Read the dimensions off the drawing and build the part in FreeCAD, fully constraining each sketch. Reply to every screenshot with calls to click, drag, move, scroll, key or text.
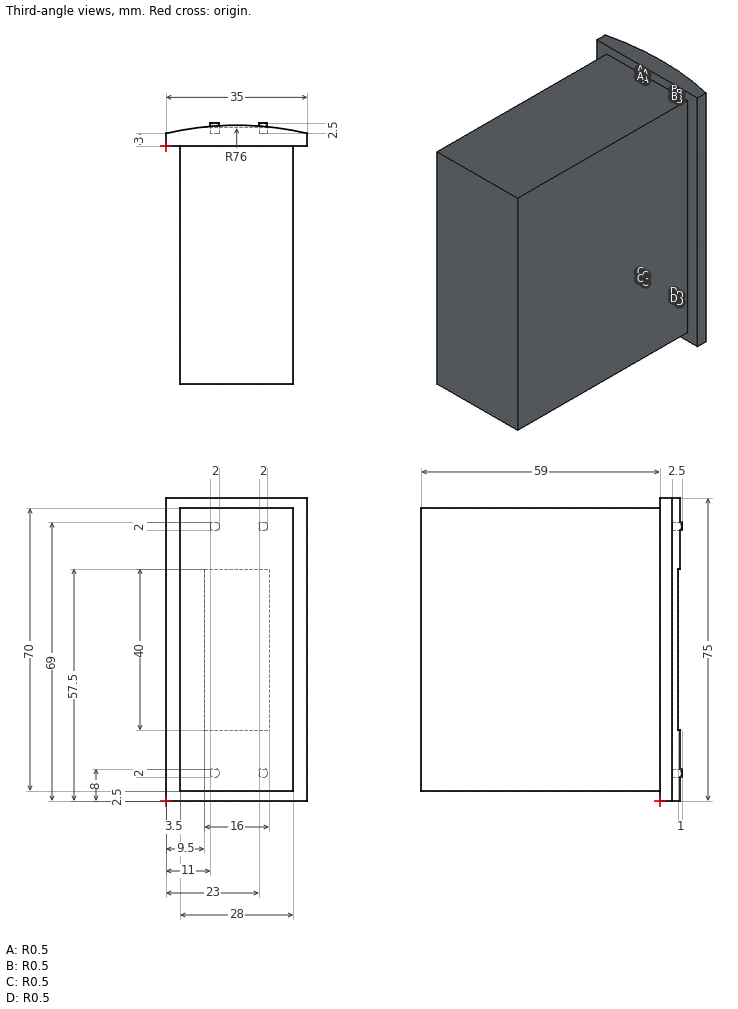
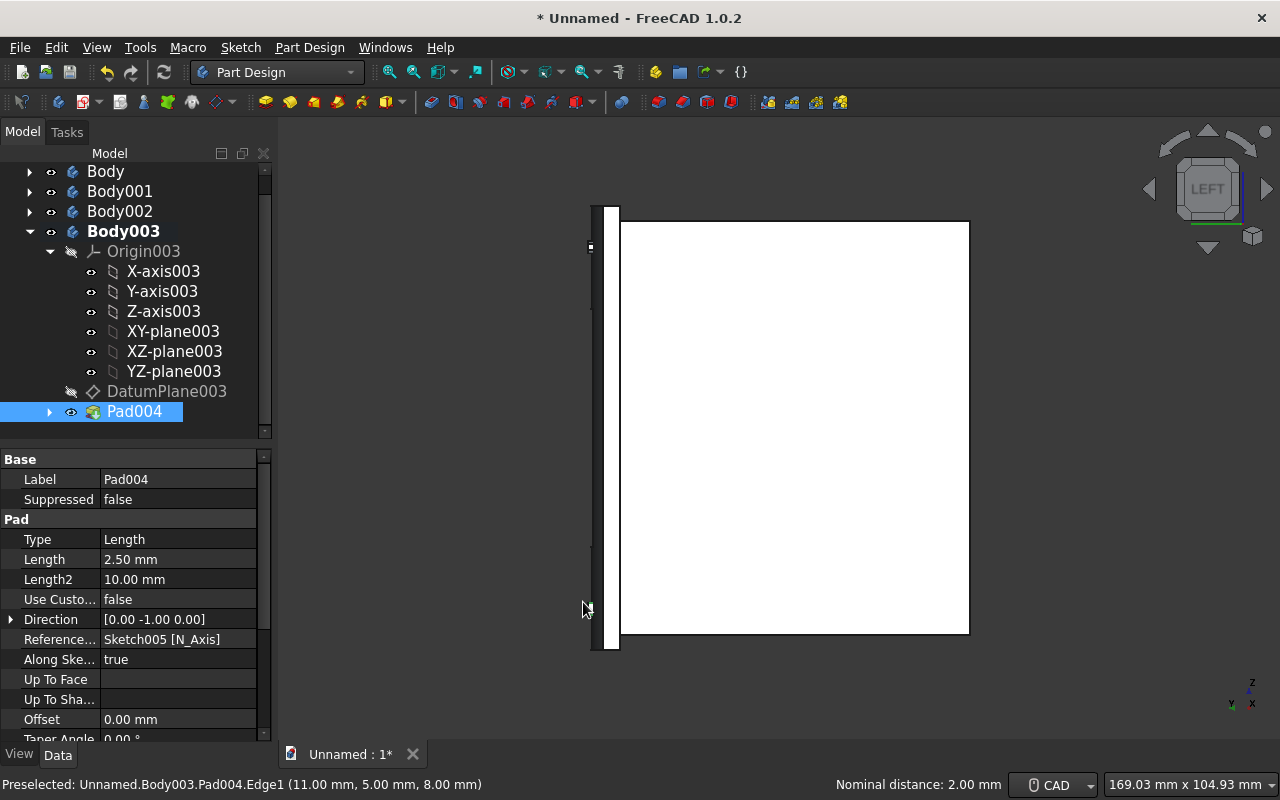
key(v)
key(3)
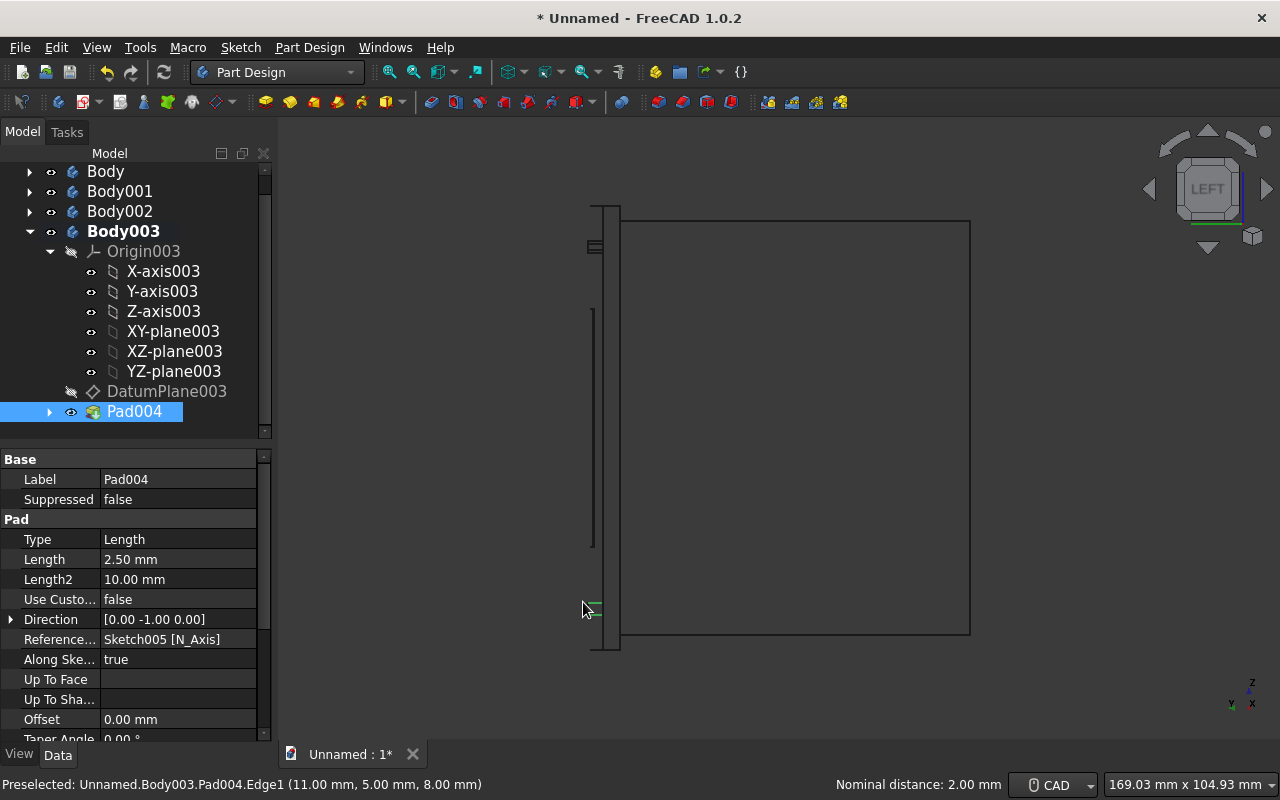
key(0)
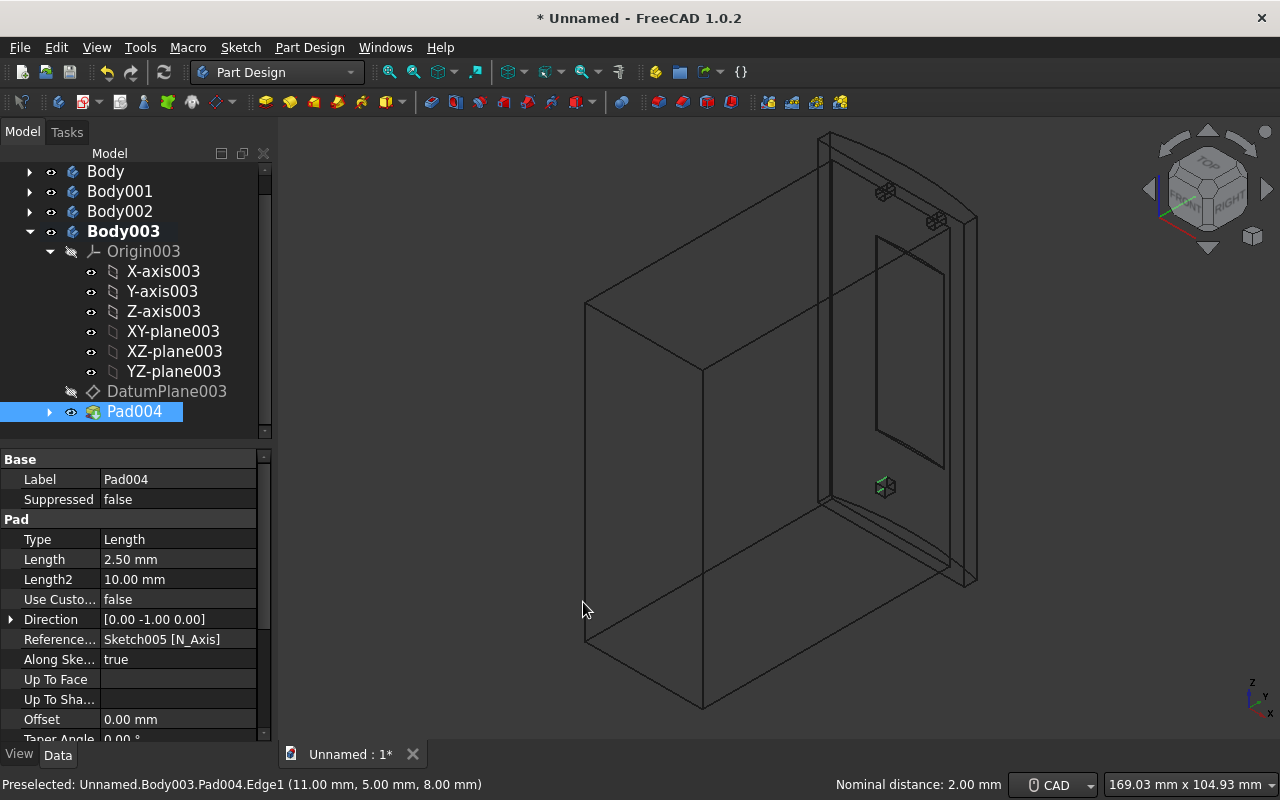
click(390, 72)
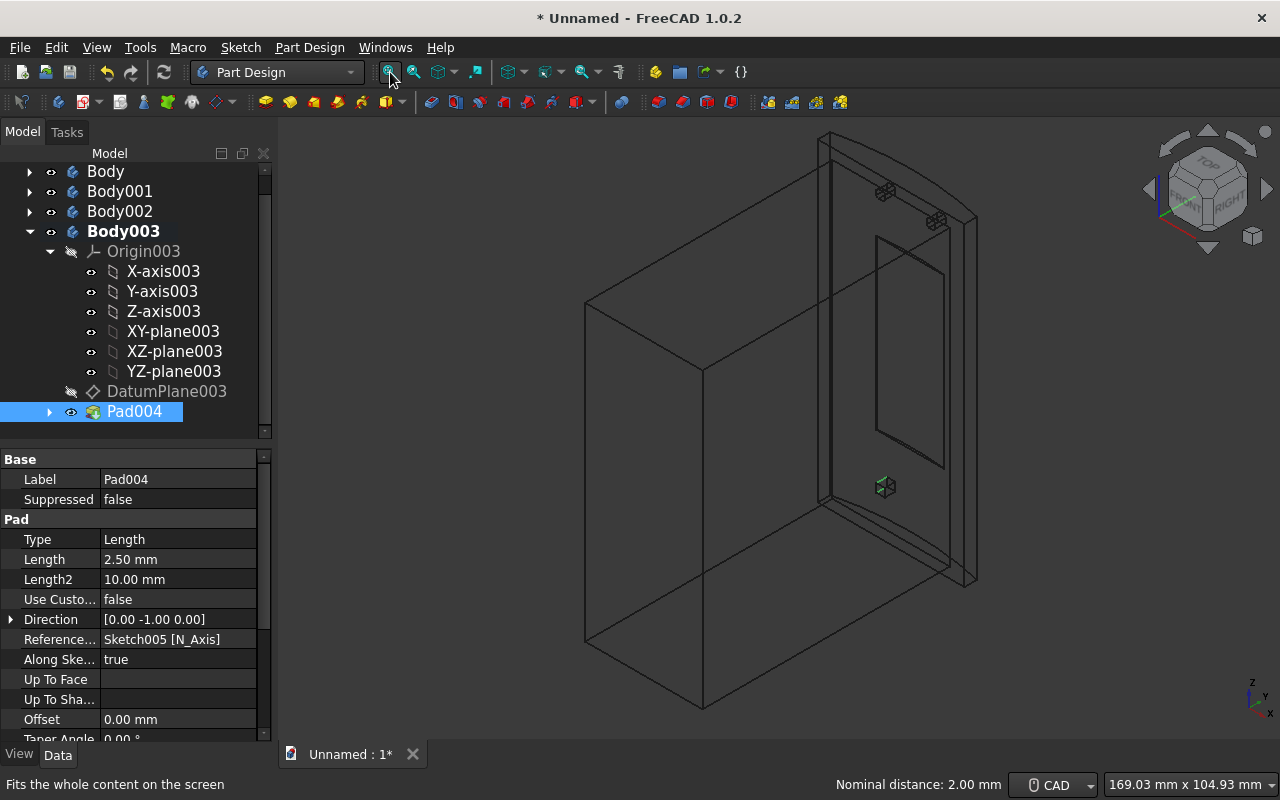
click(891, 483, ctrl)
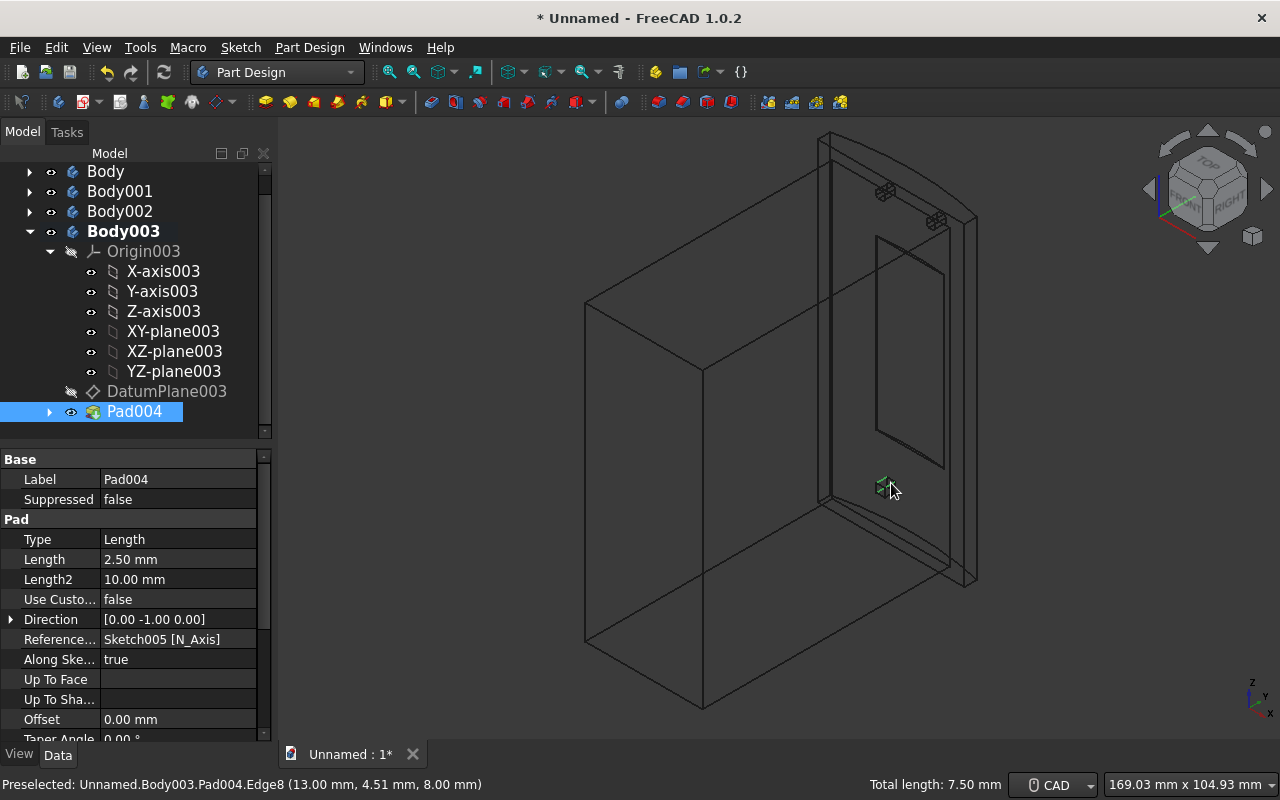
click(891, 493, ctrl)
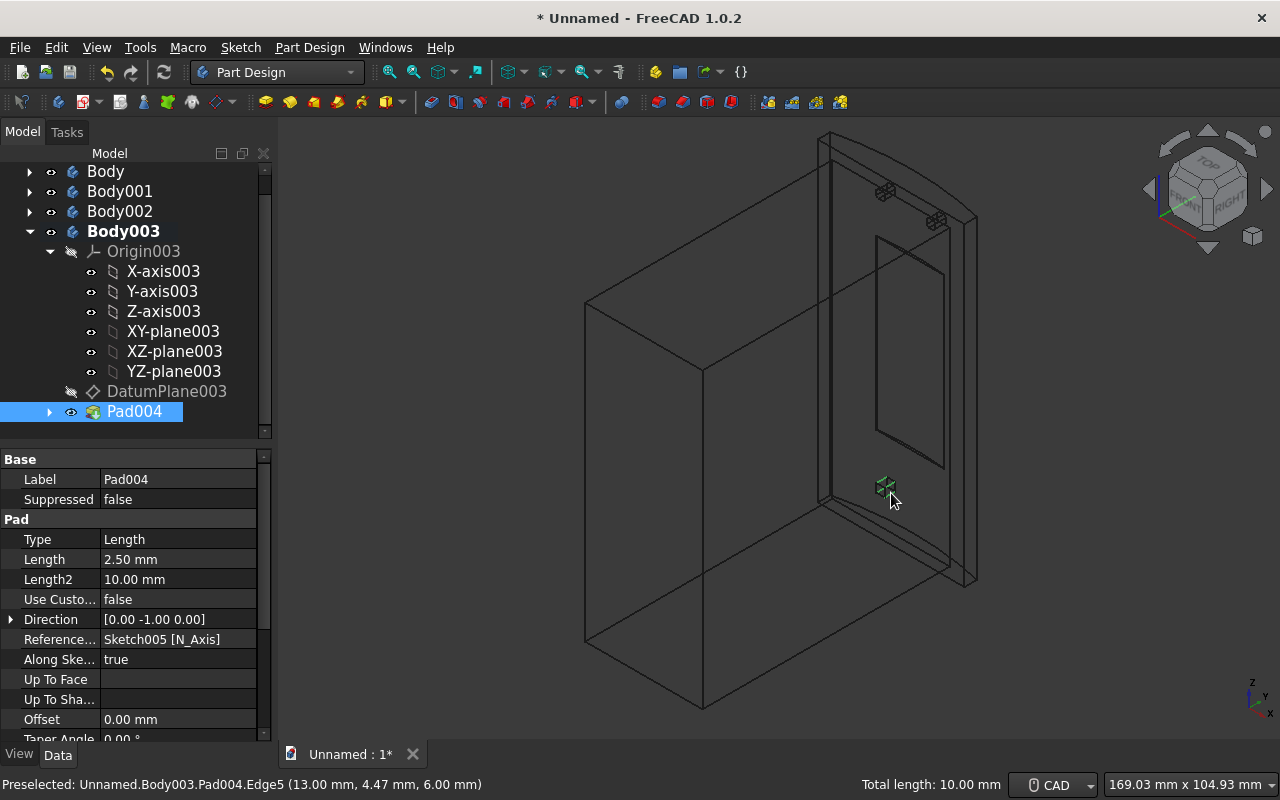
key(v)
key(1)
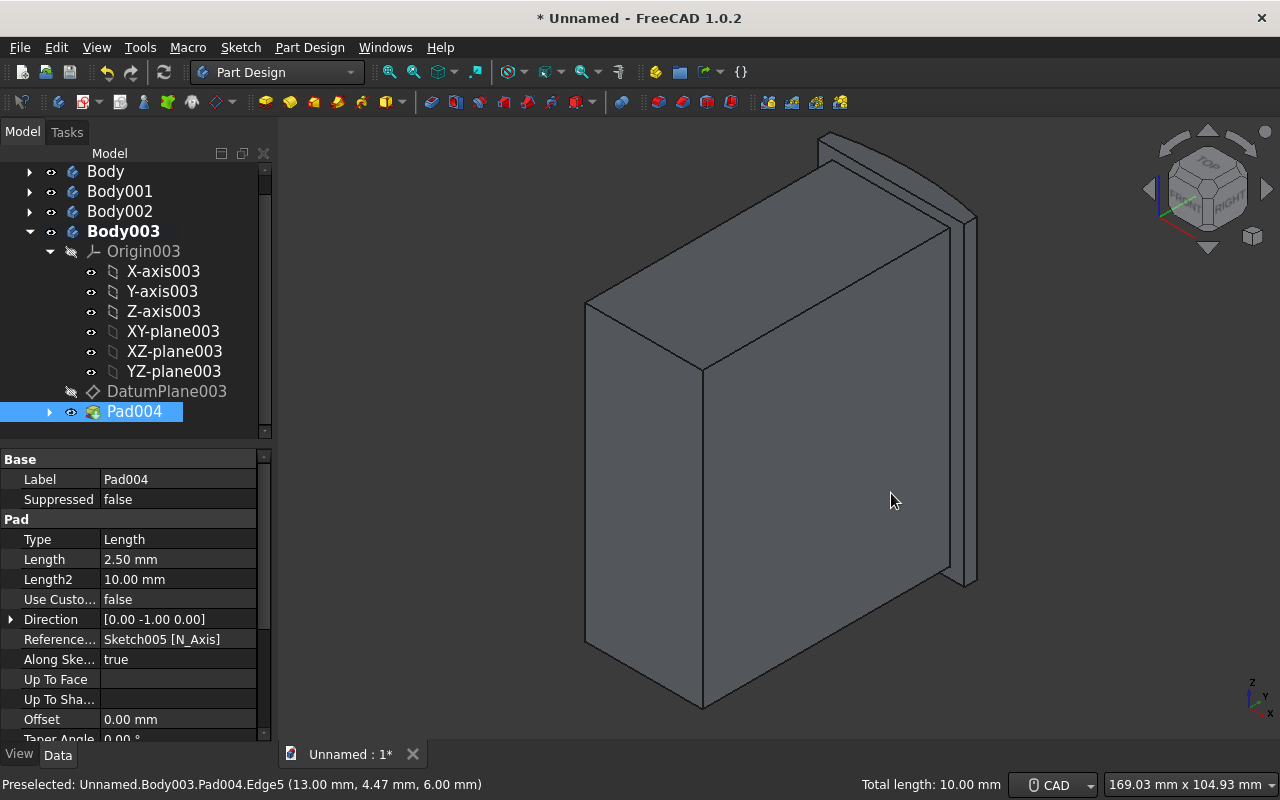
click(660, 102)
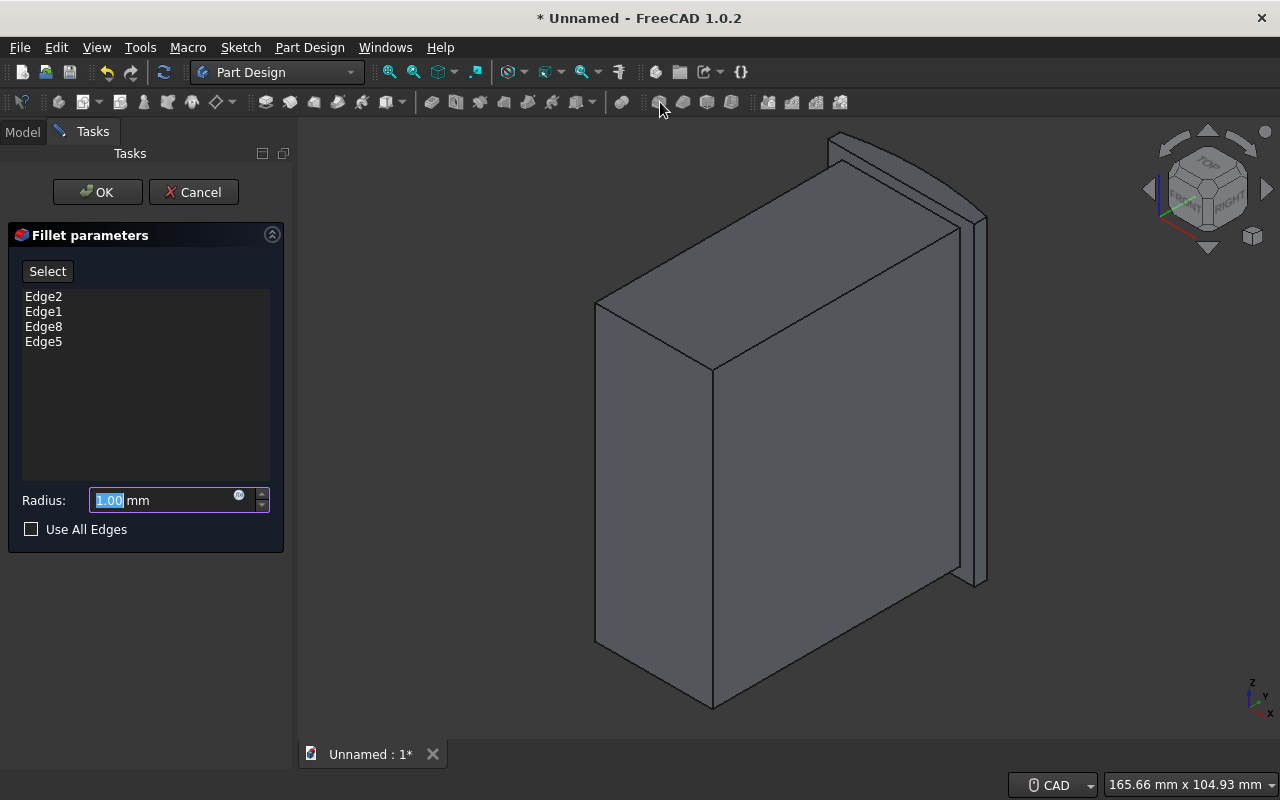
text(0.5)
key(Tab)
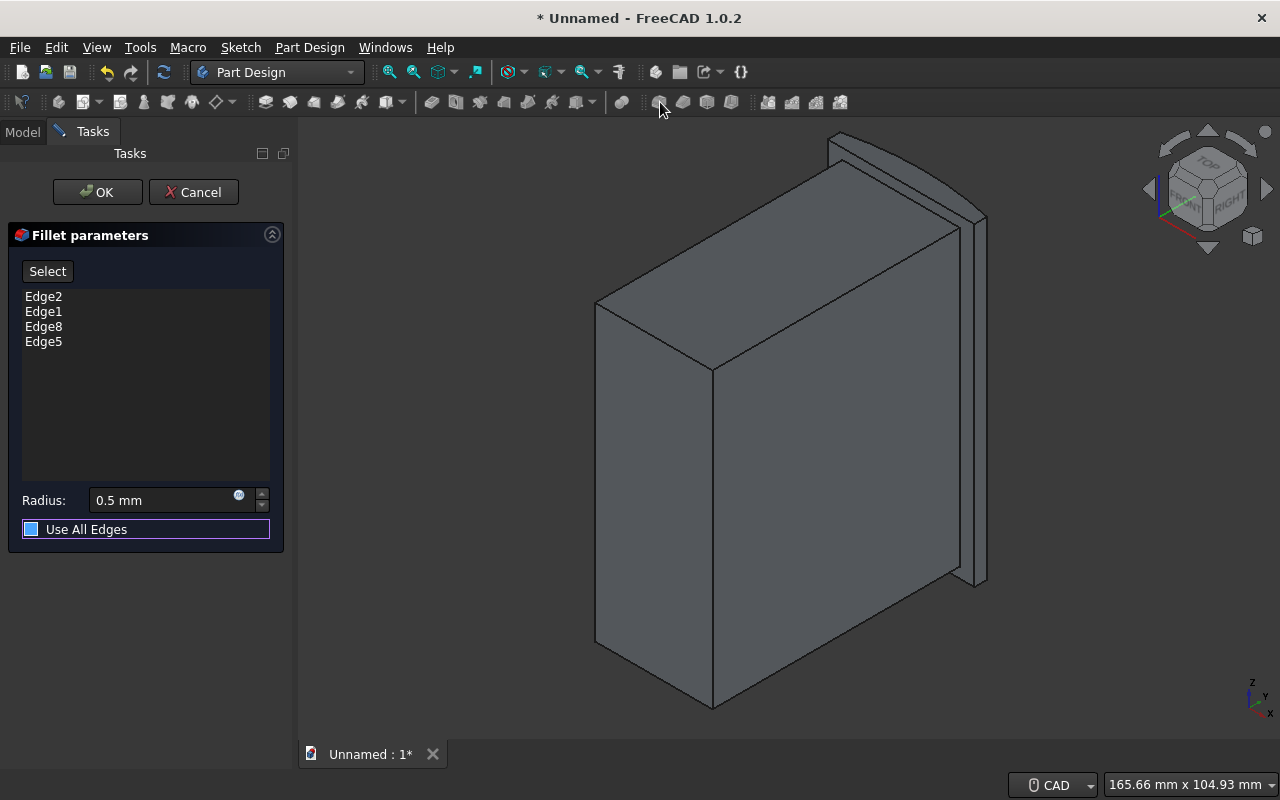
click(98, 192)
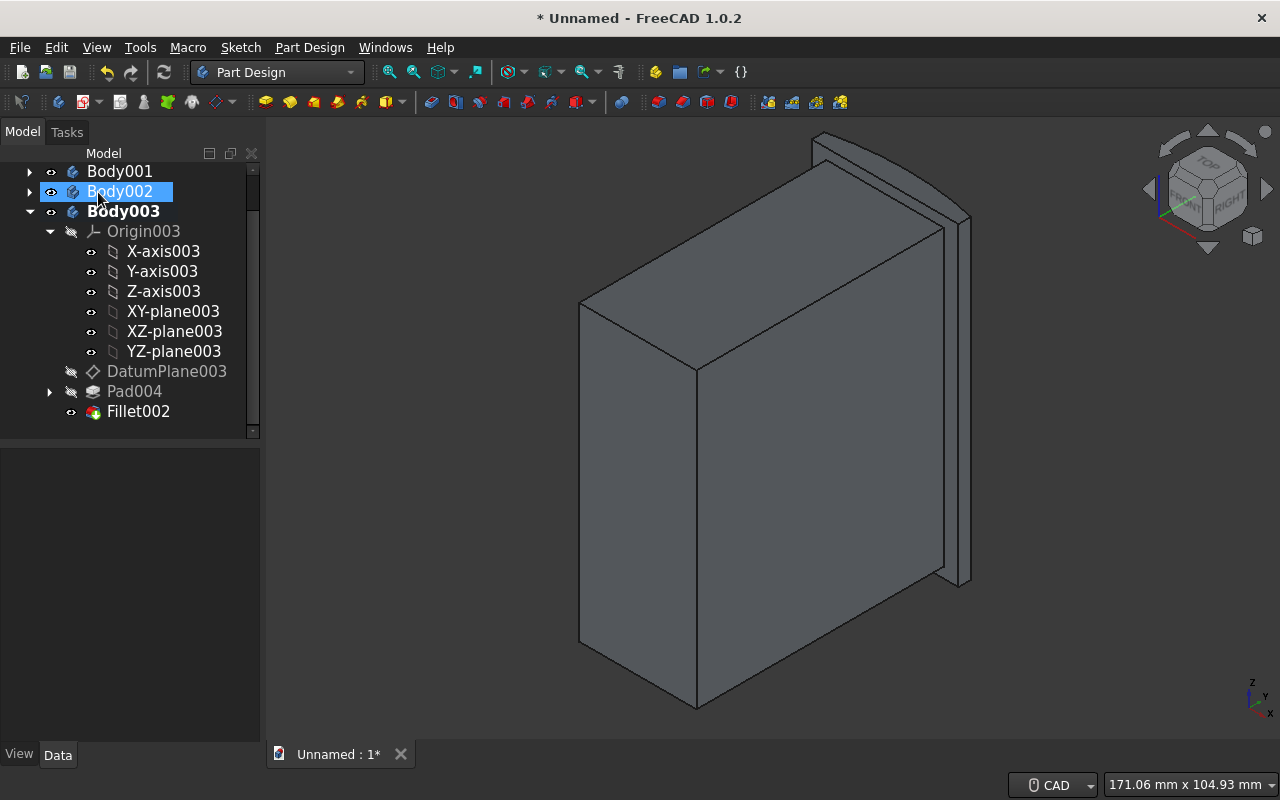
click(390, 72)